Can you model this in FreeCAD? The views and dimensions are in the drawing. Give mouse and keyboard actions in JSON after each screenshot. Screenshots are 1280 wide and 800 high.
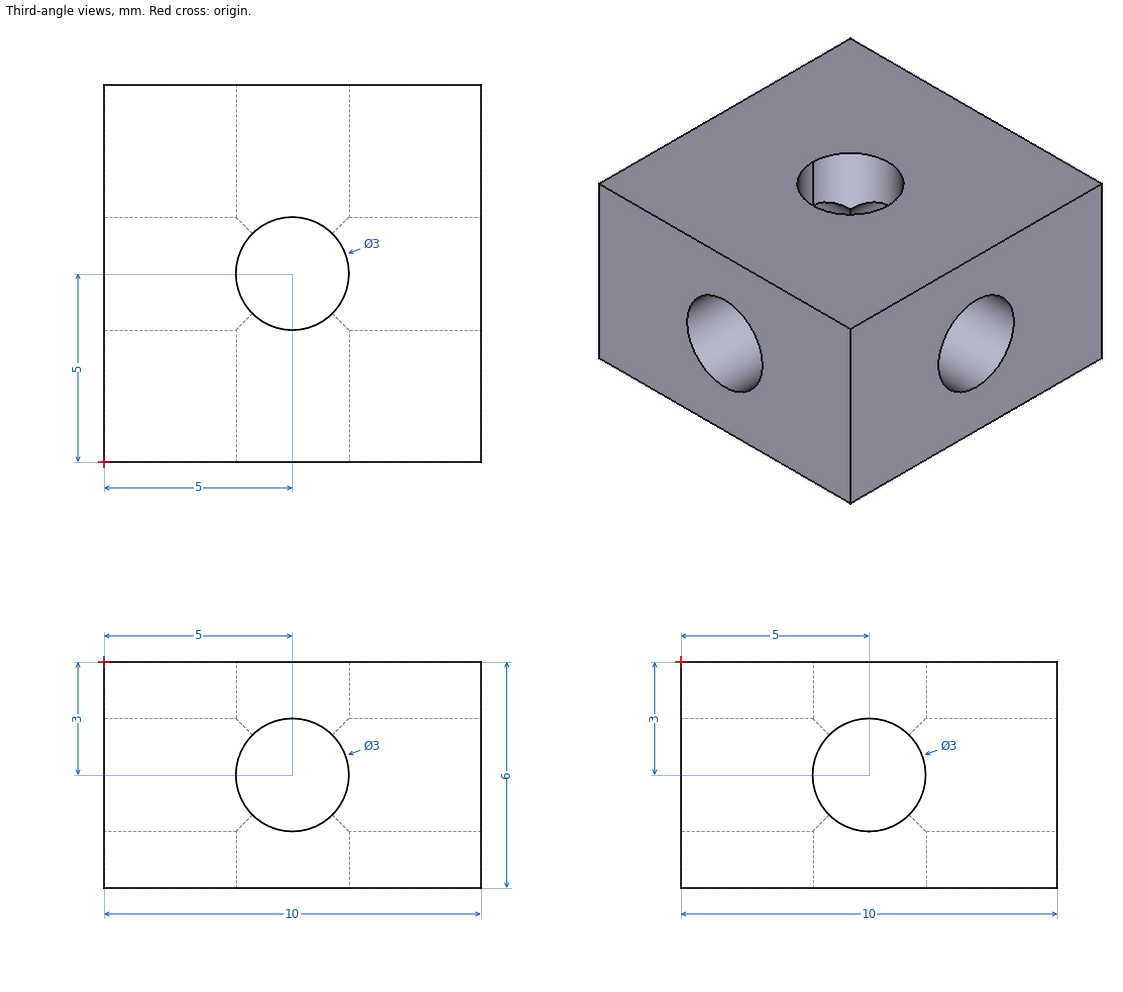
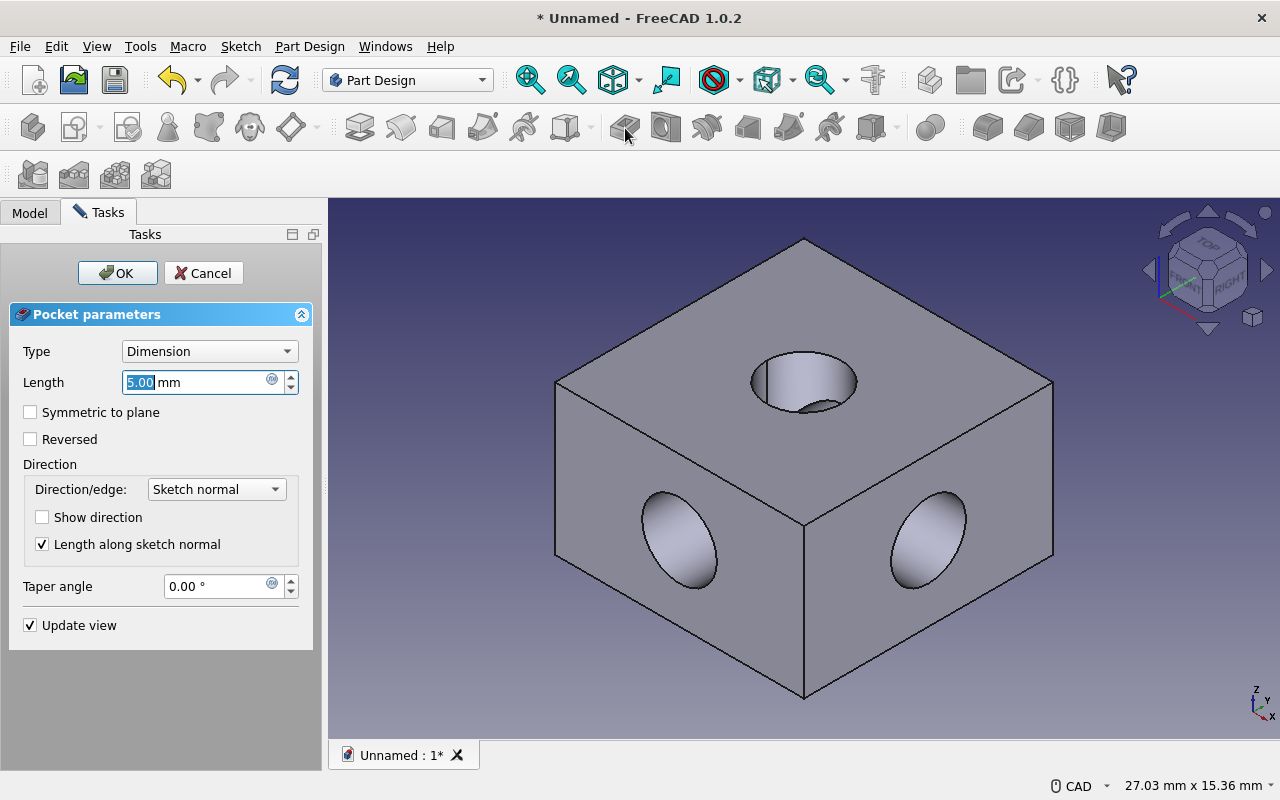
{"action": "left_click", "coordinate": [210, 352]}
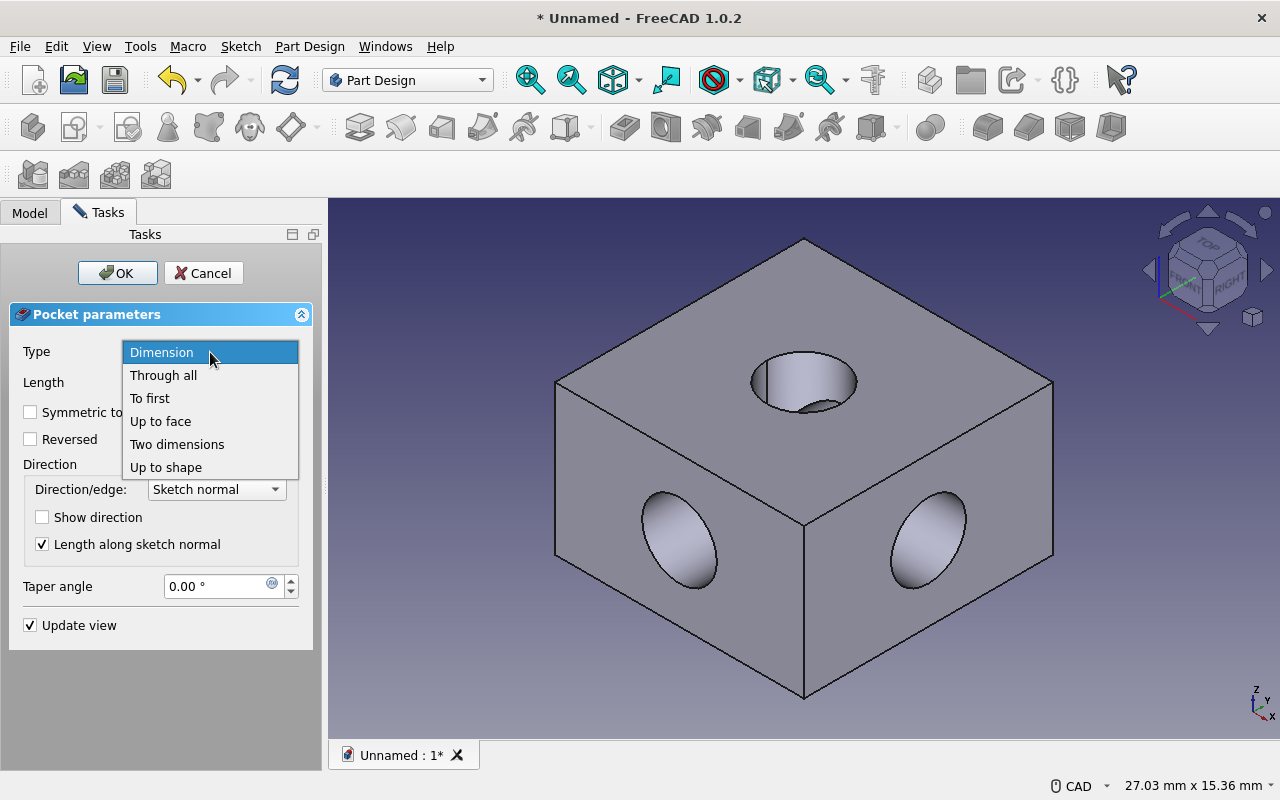
{"action": "left_click", "coordinate": [208, 376]}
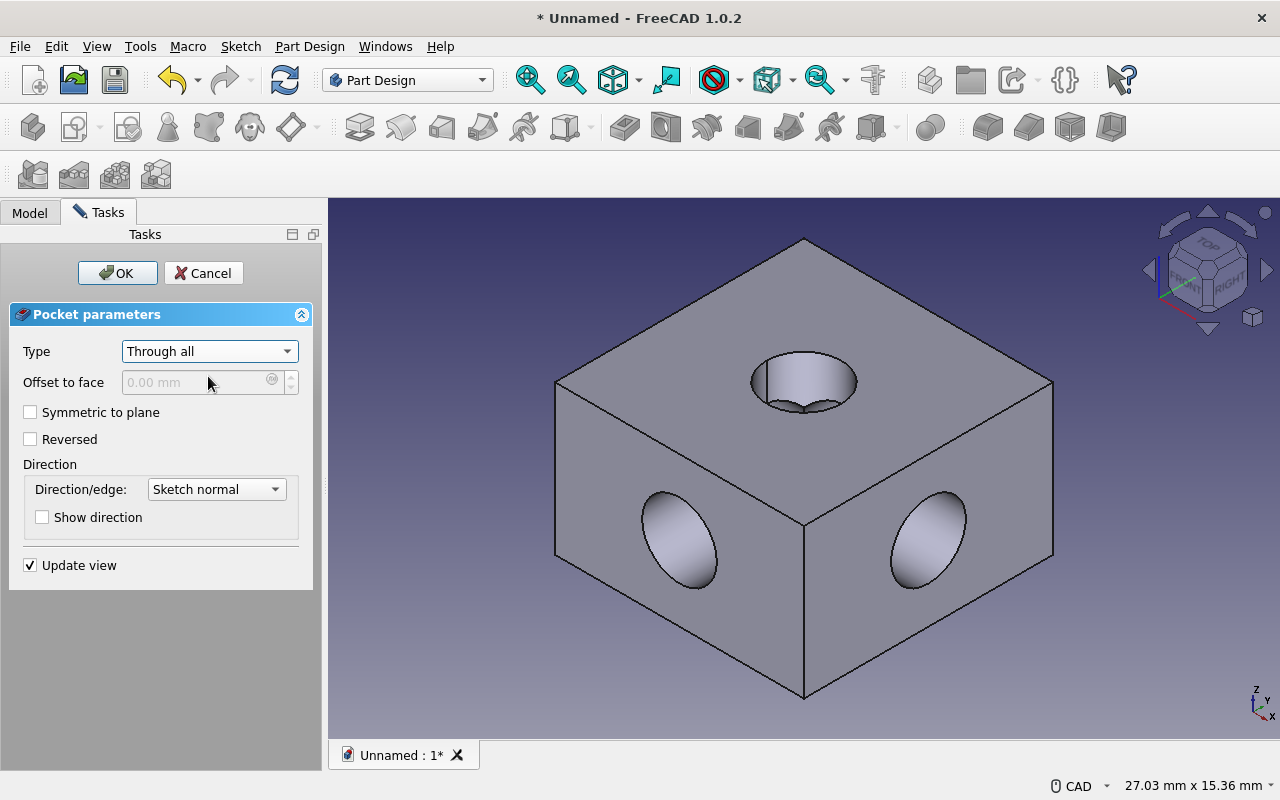
{"action": "left_click", "coordinate": [118, 273]}